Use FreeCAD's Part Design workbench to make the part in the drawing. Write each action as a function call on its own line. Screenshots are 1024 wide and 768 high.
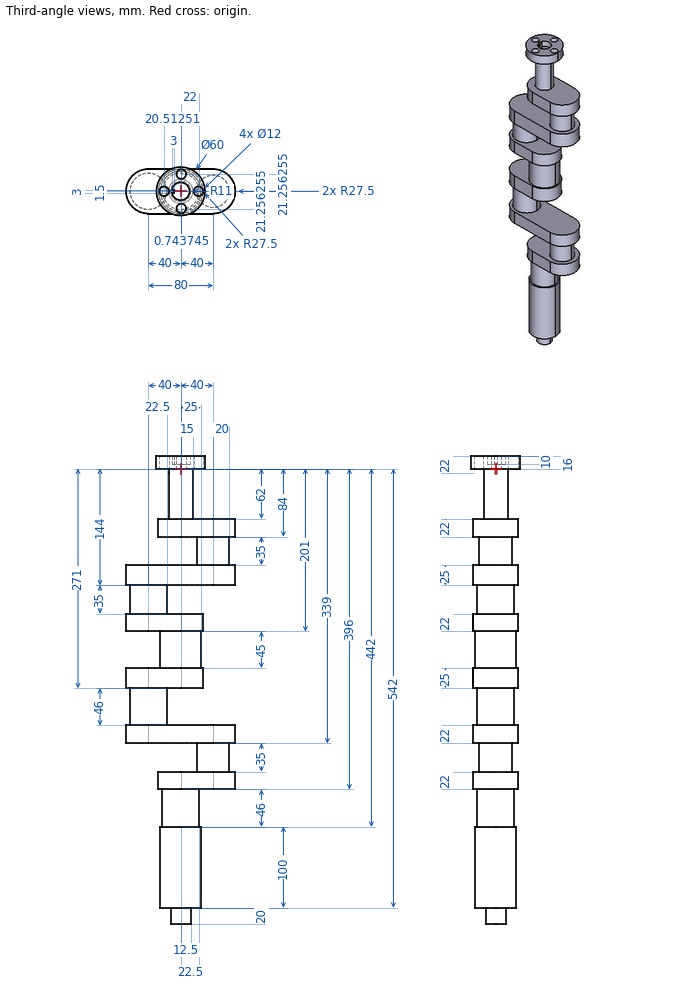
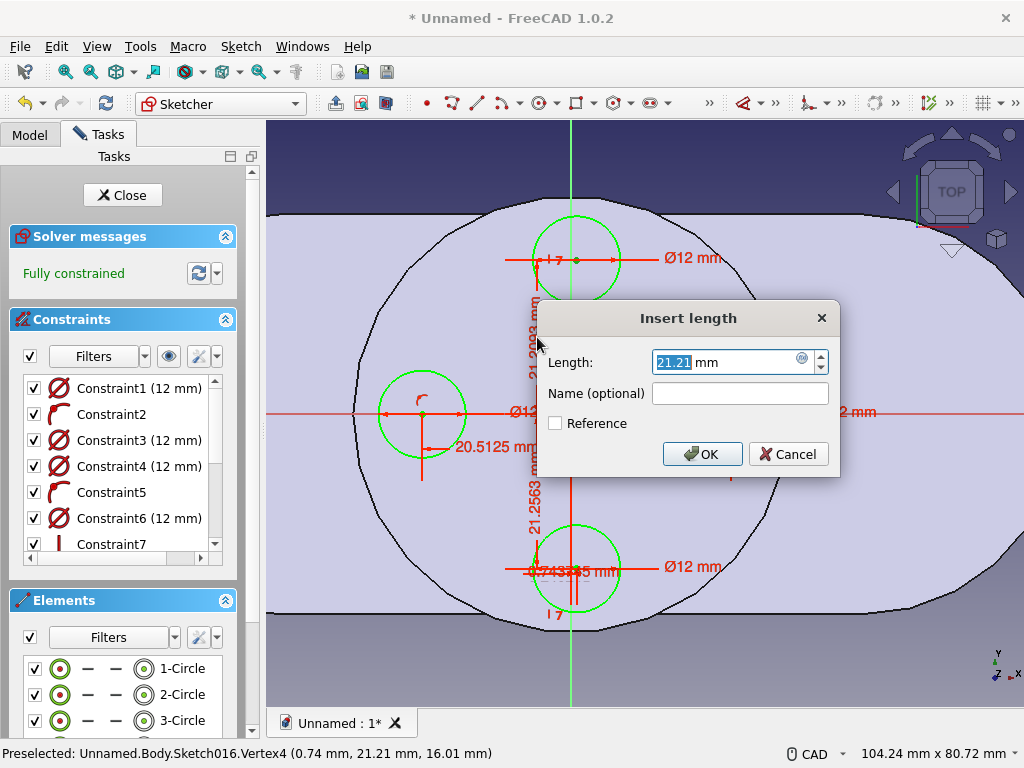
text(21.256255)
key(Return)
key(Escape)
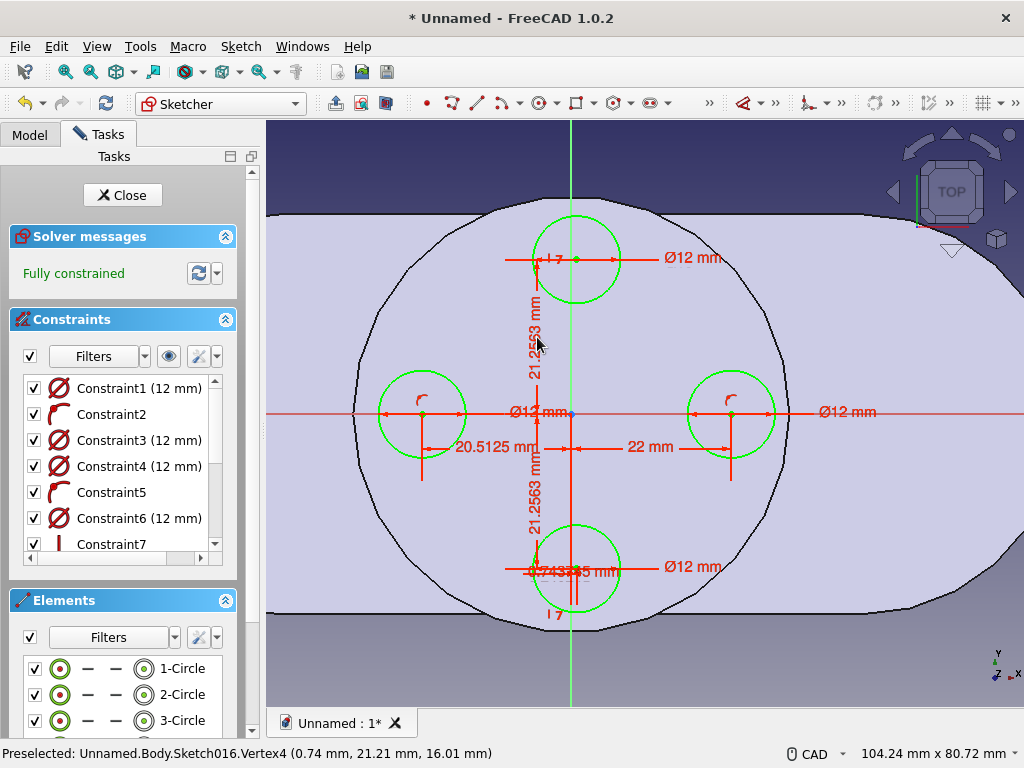
click(123, 195)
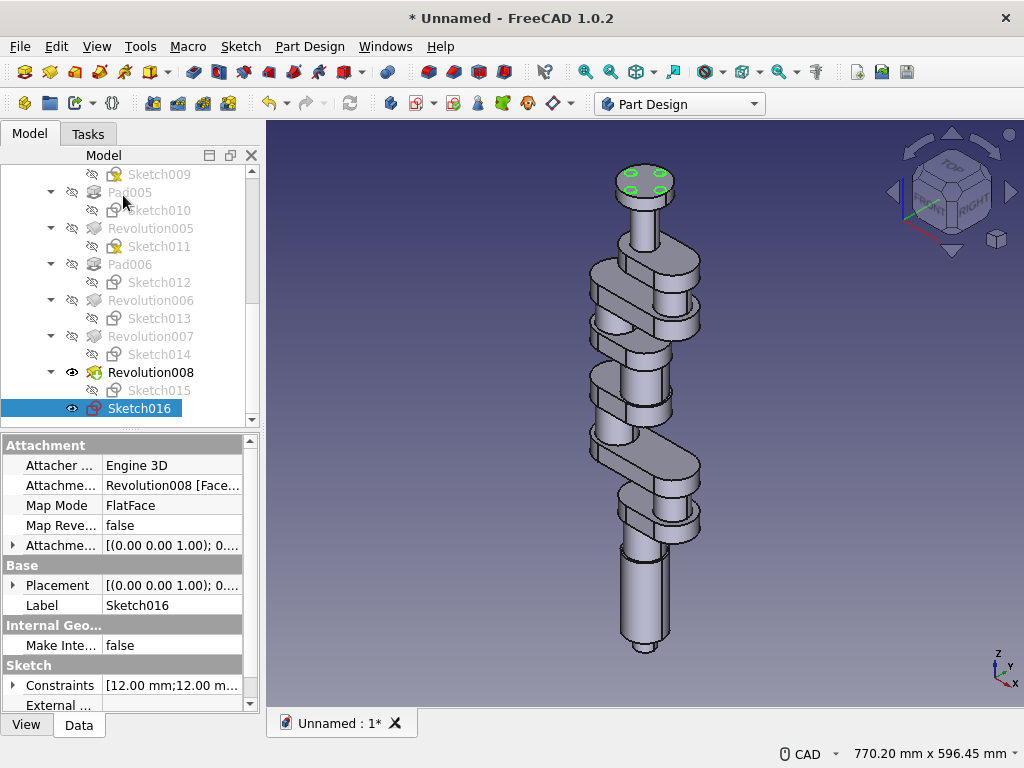
click(194, 72)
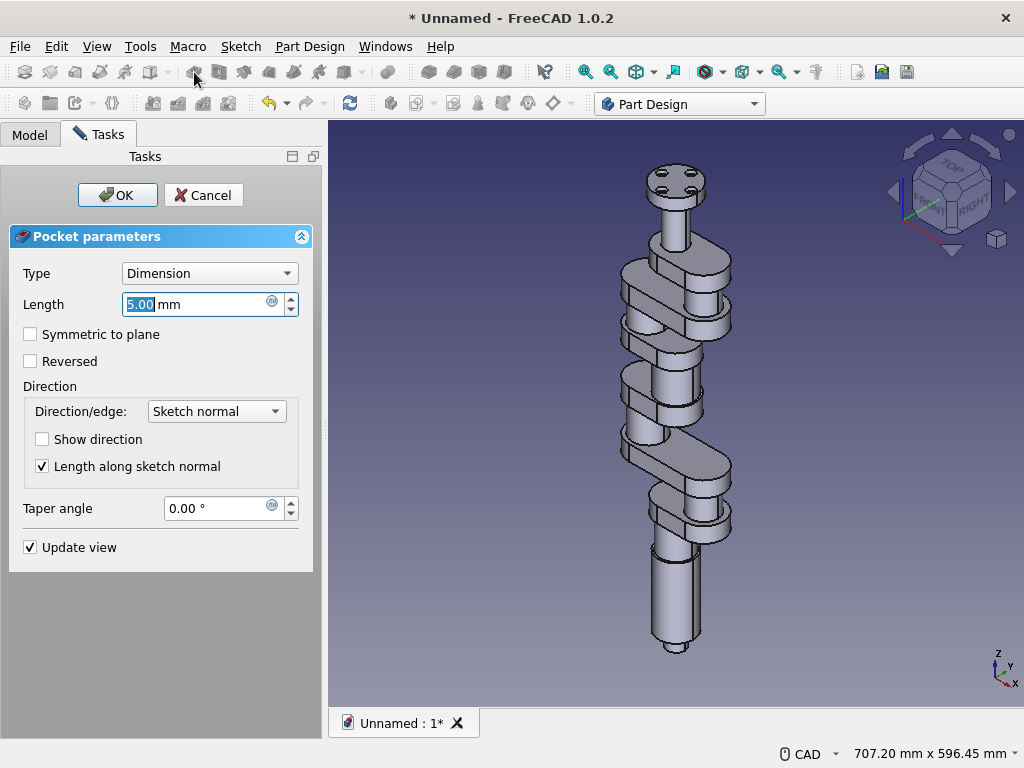
text(22)
key(Tab)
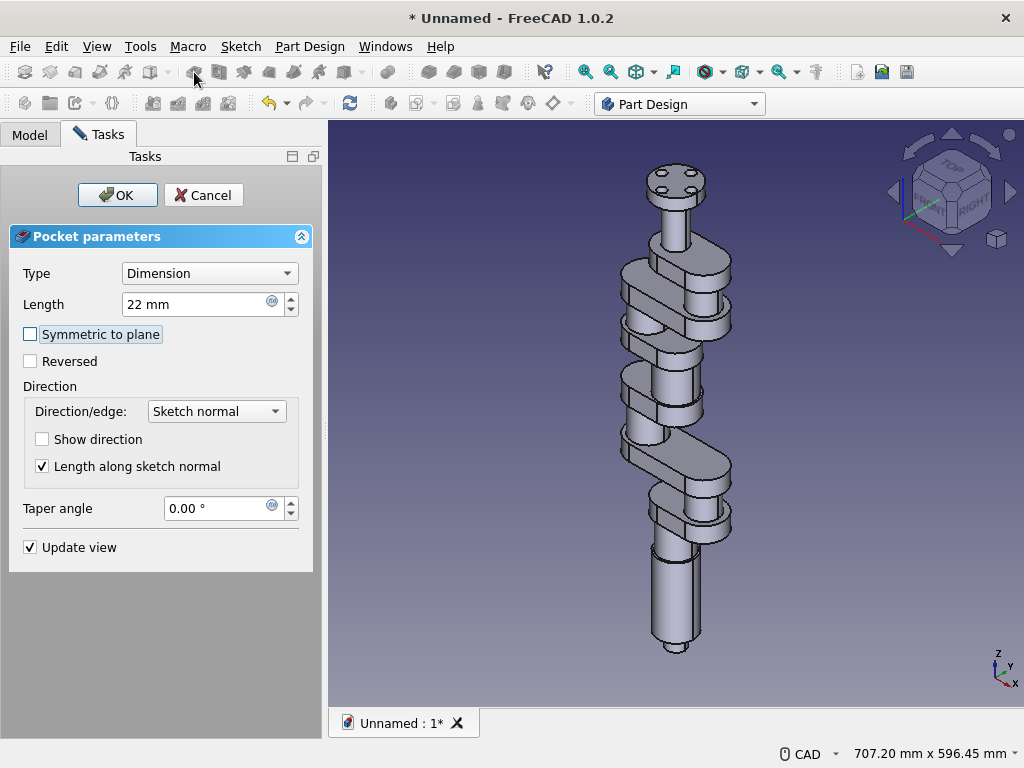
click(118, 195)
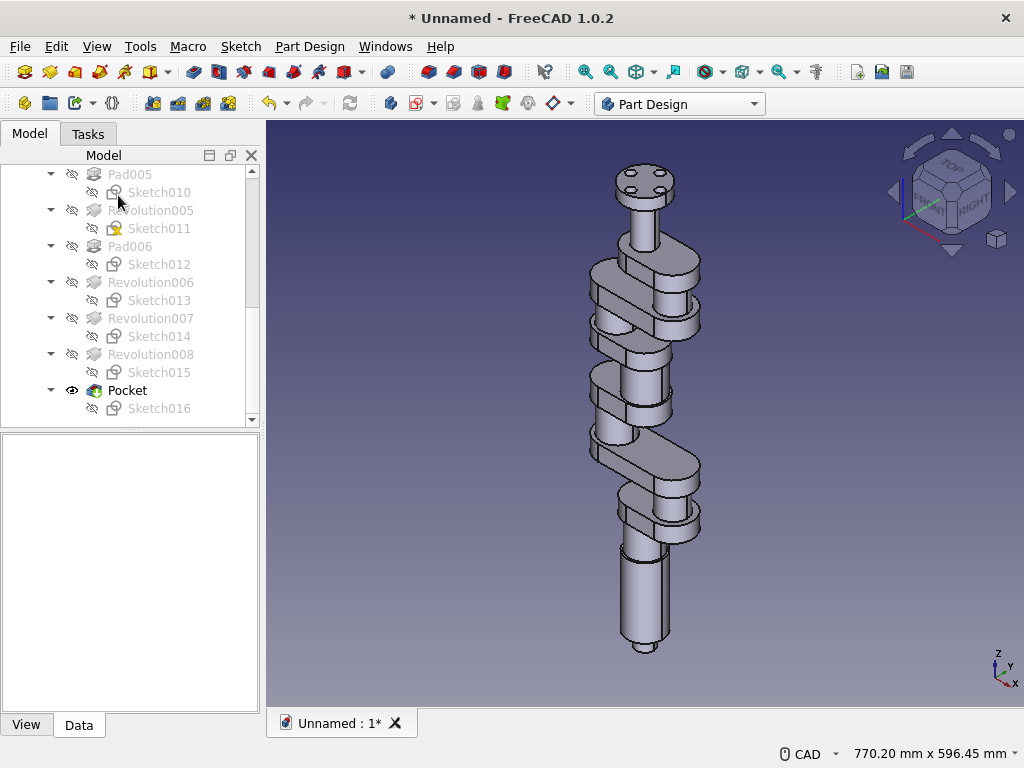
click(645, 180)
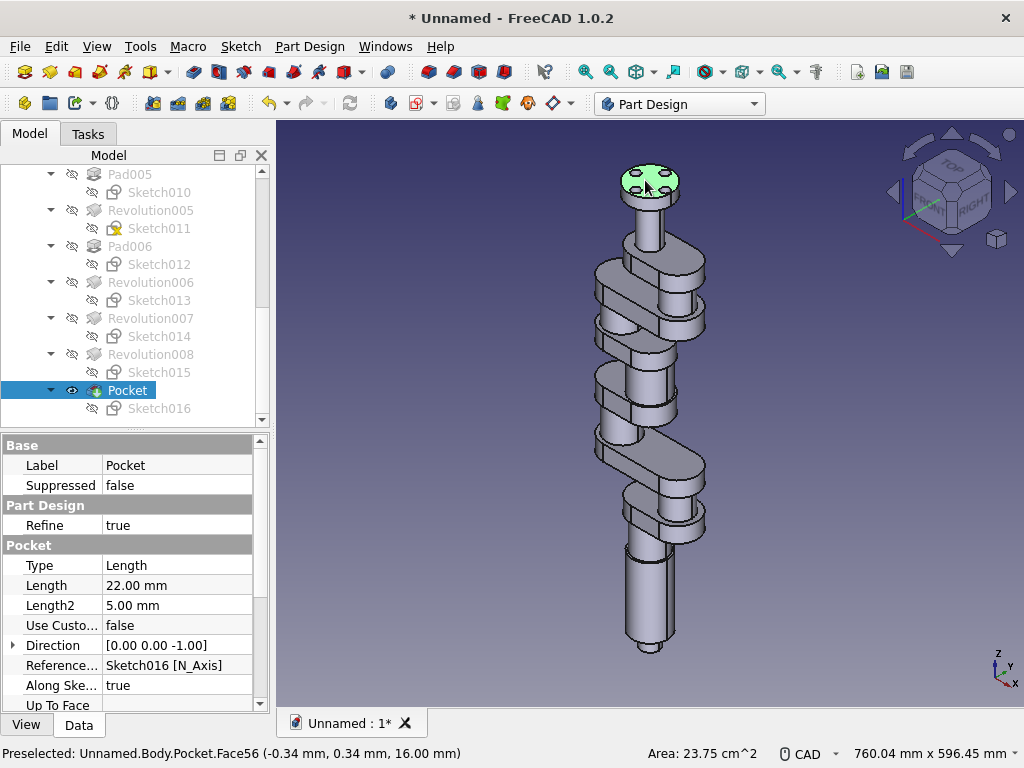
click(416, 104)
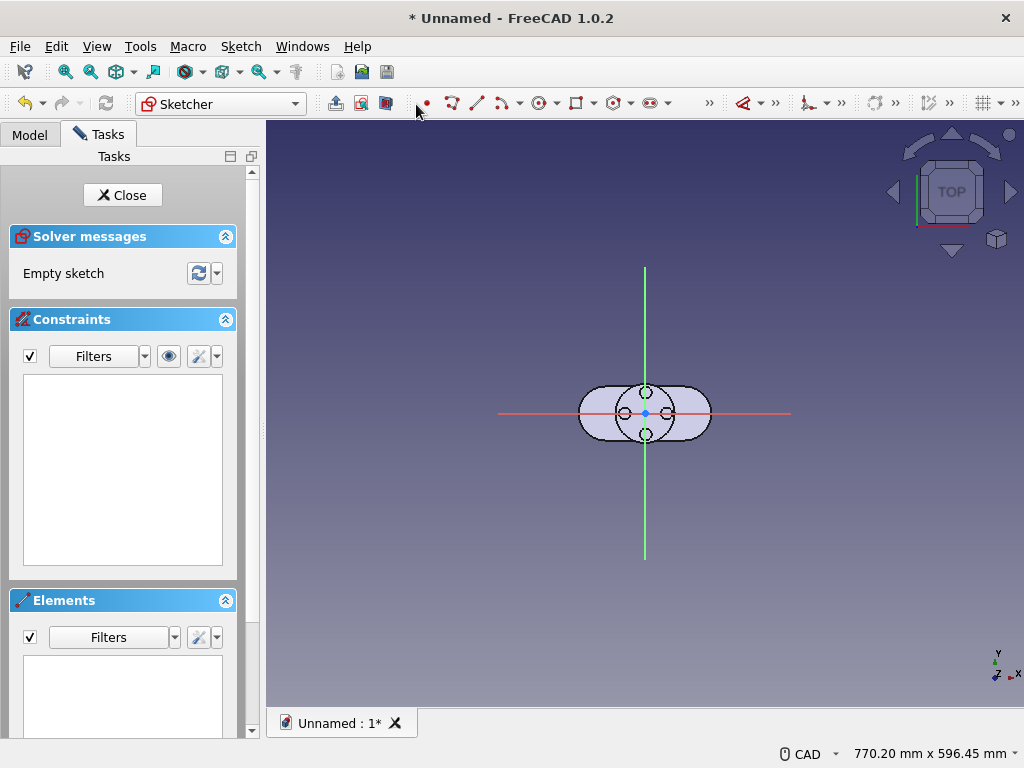
scroll(649, 413, up, 15)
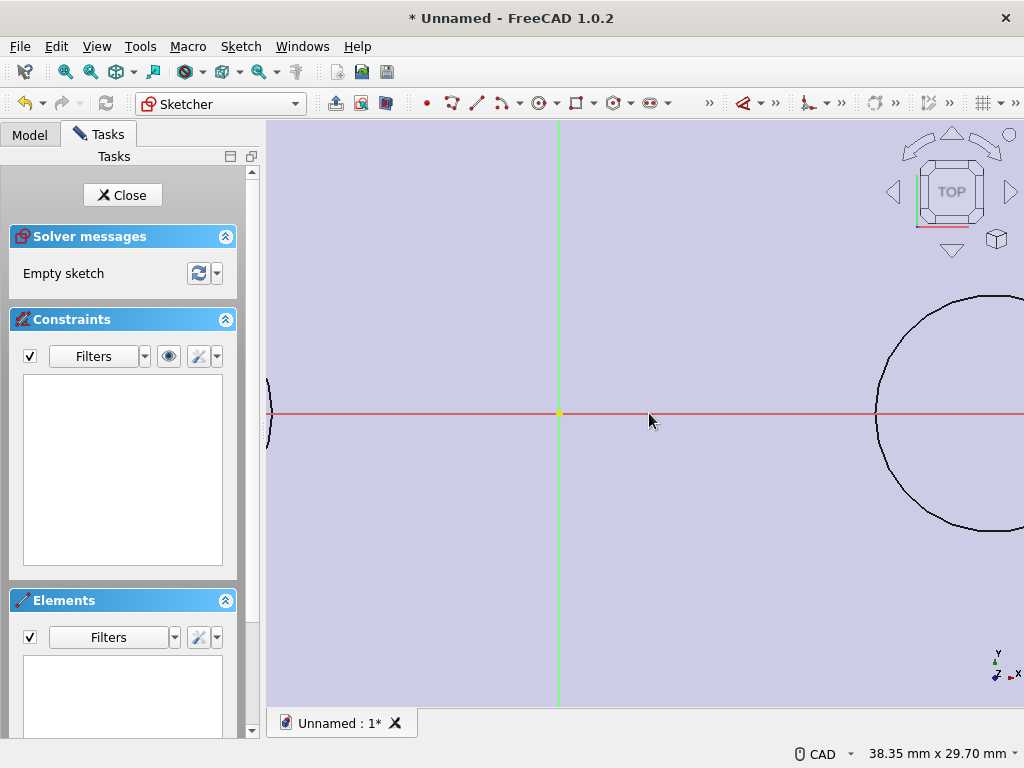
key(g)
key(m)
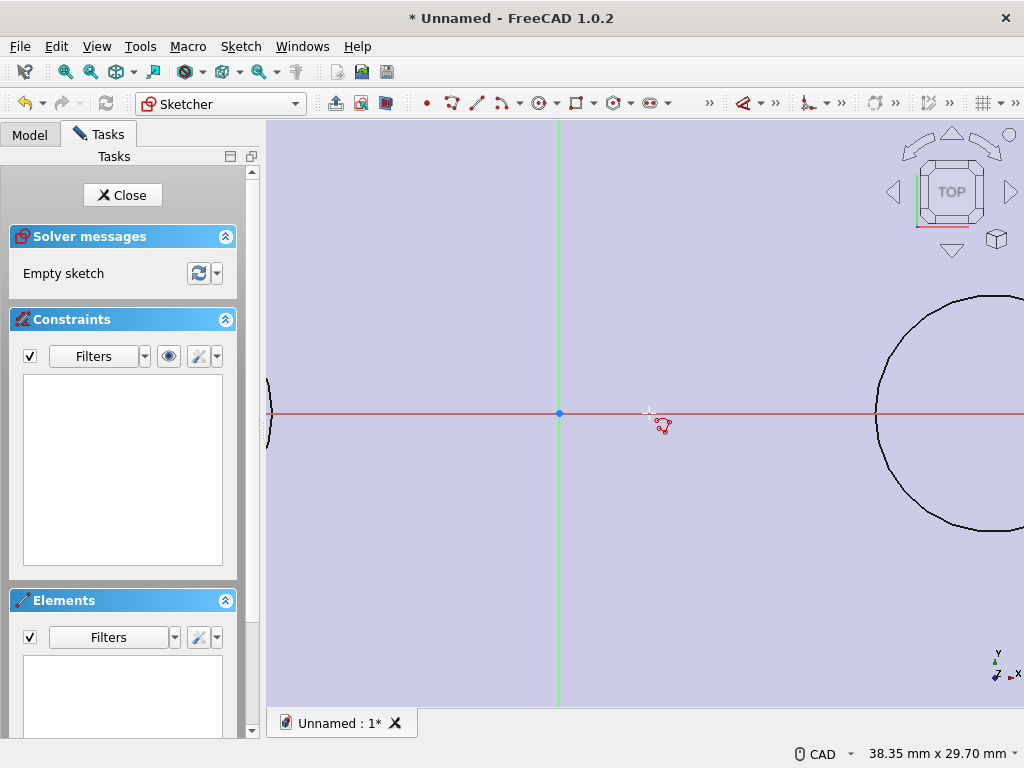
click(344, 384)
click(403, 384)
click(403, 443)
click(344, 443)
right_click(344, 443)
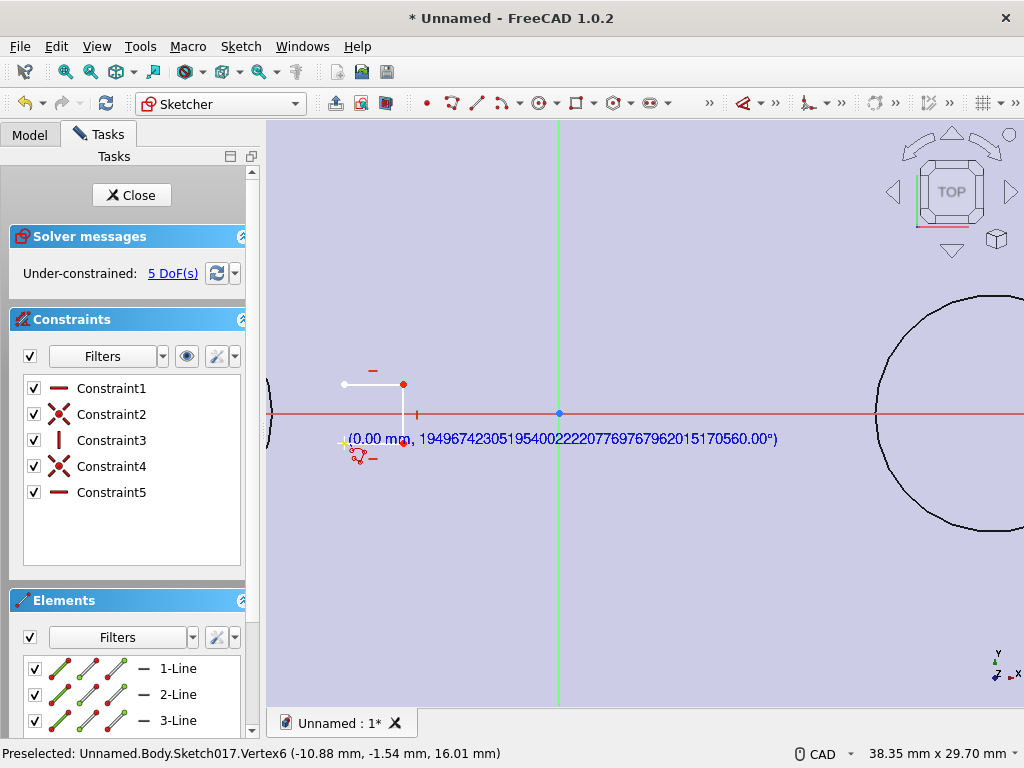
key(g)
key(3)
key(a)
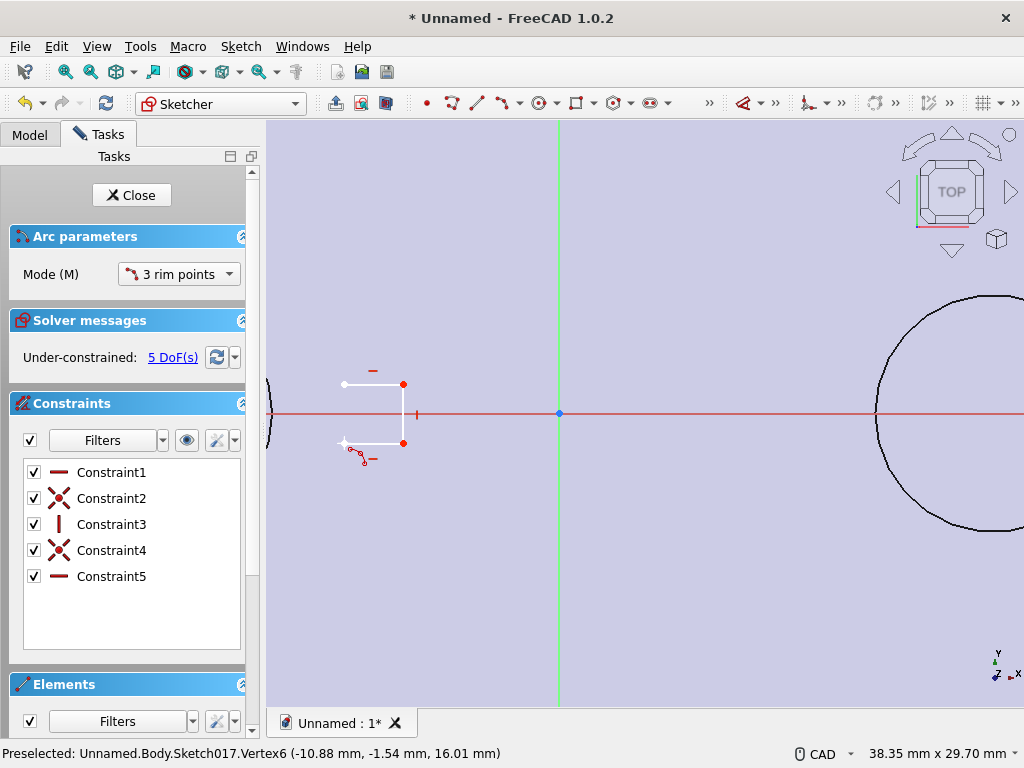
click(344, 444)
click(344, 385)
click(738, 536)
key(Escape)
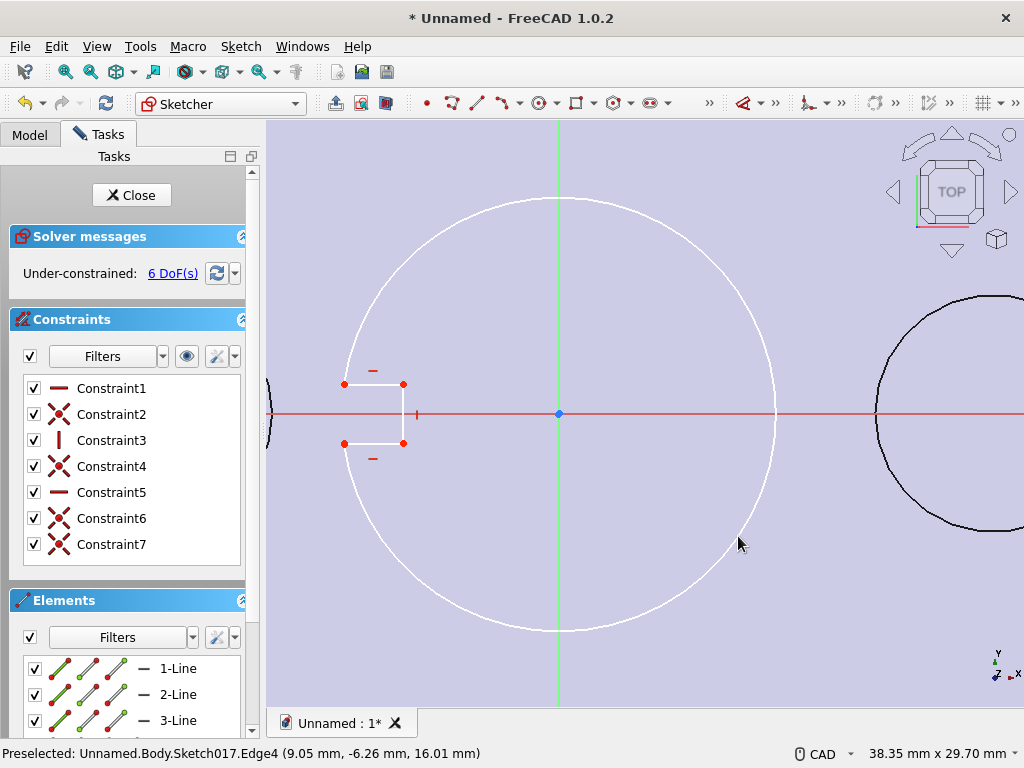
drag(549, 403, 569, 425)